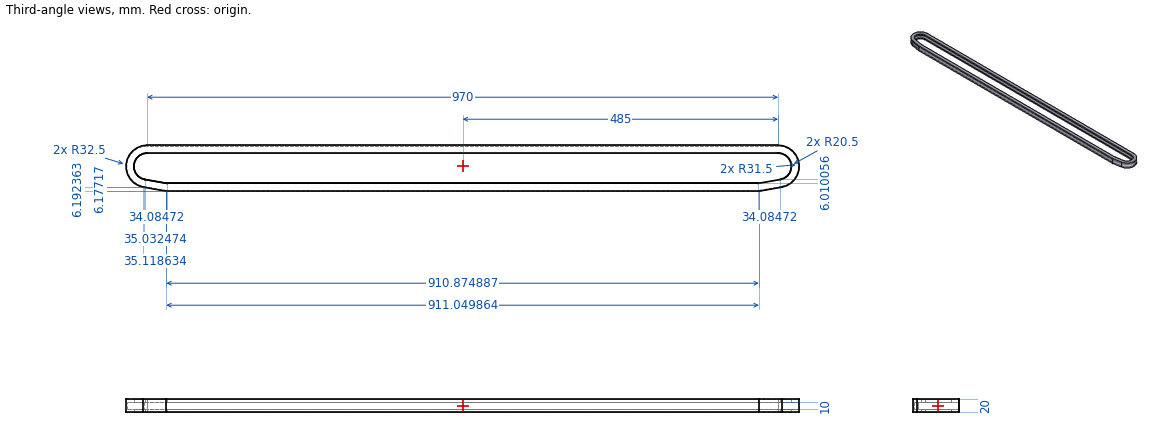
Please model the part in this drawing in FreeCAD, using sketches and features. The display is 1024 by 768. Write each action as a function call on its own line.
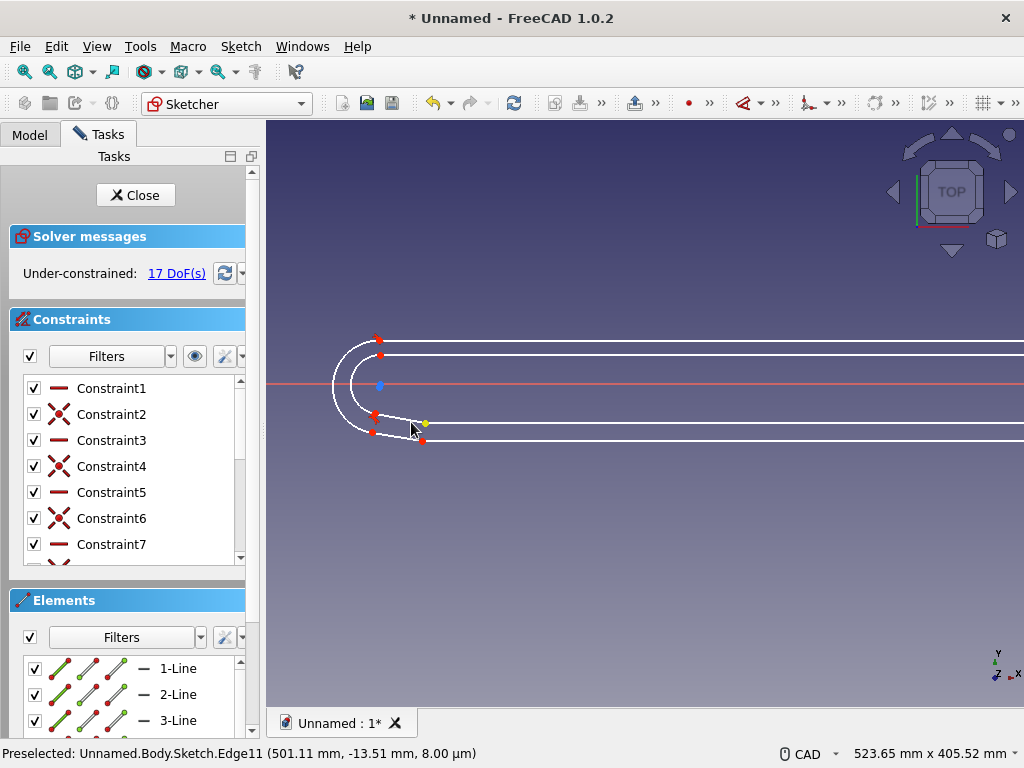
click(410, 420)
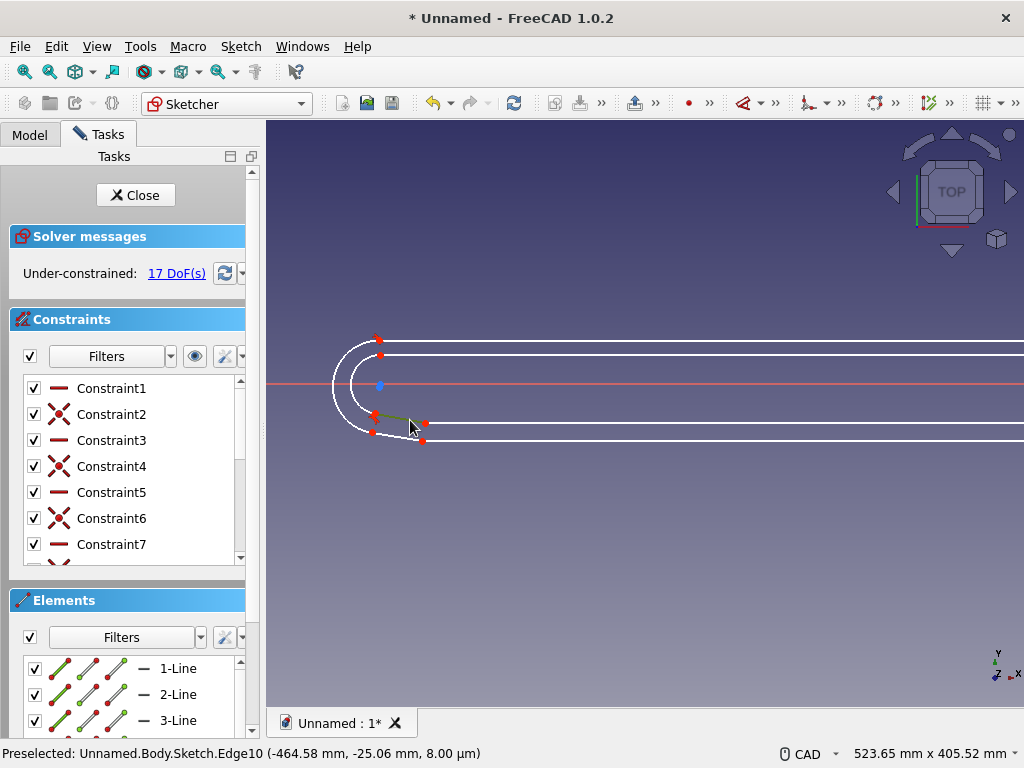
click(358, 366)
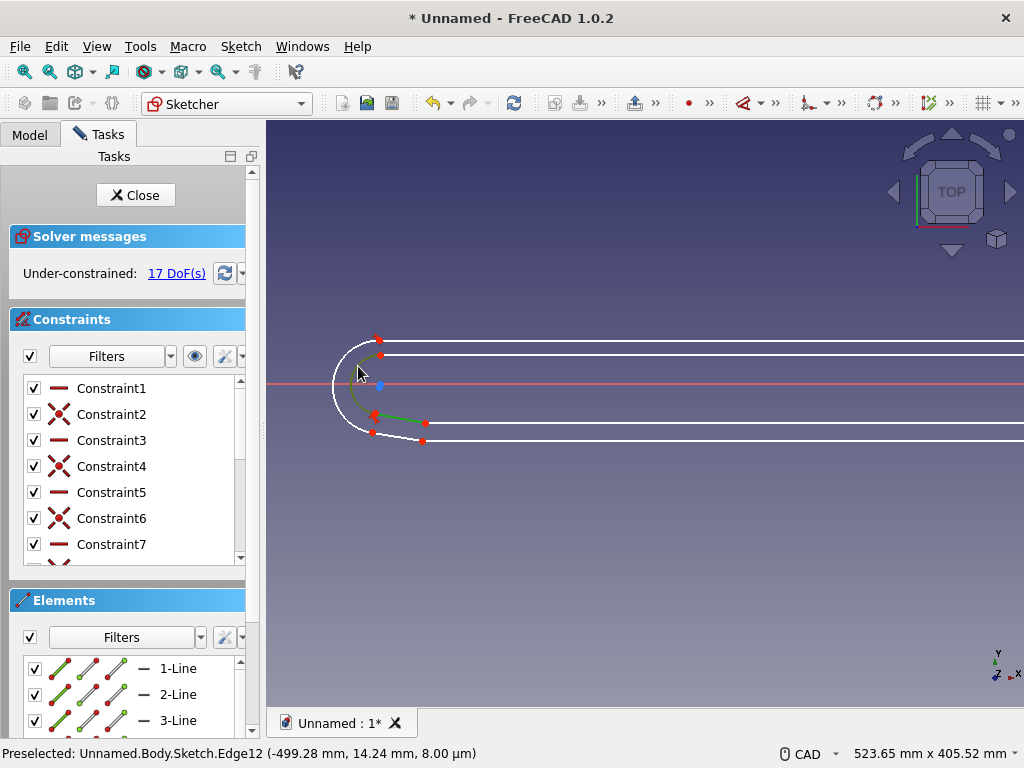
key(t)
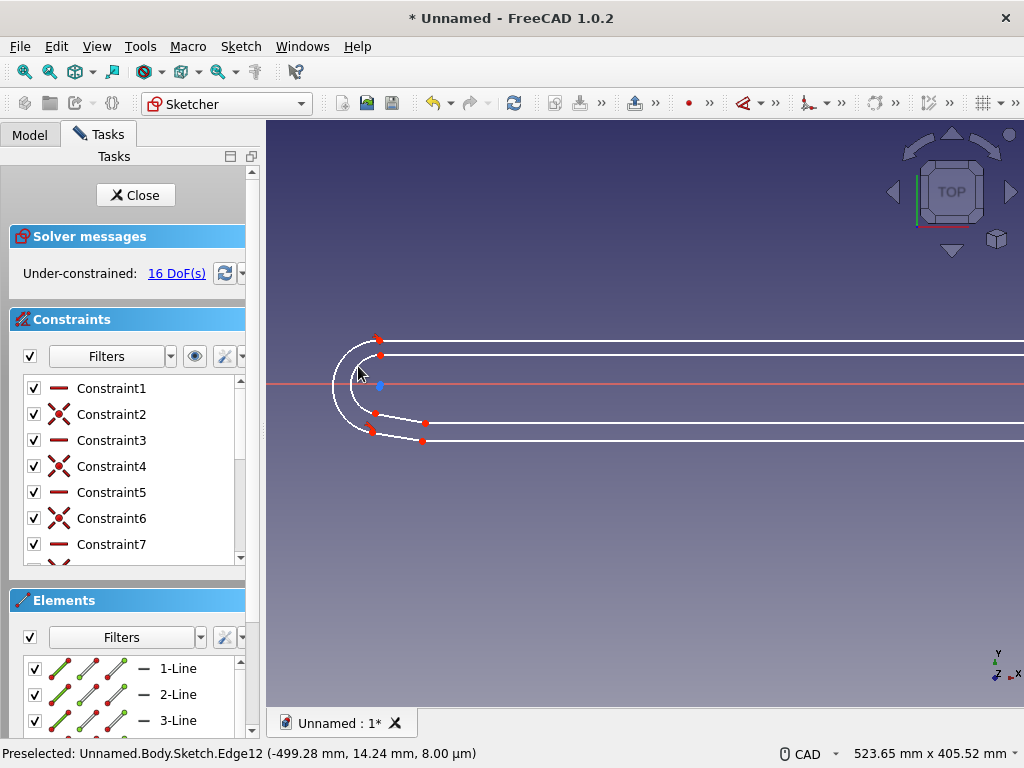
scroll(411, 422, down, 7)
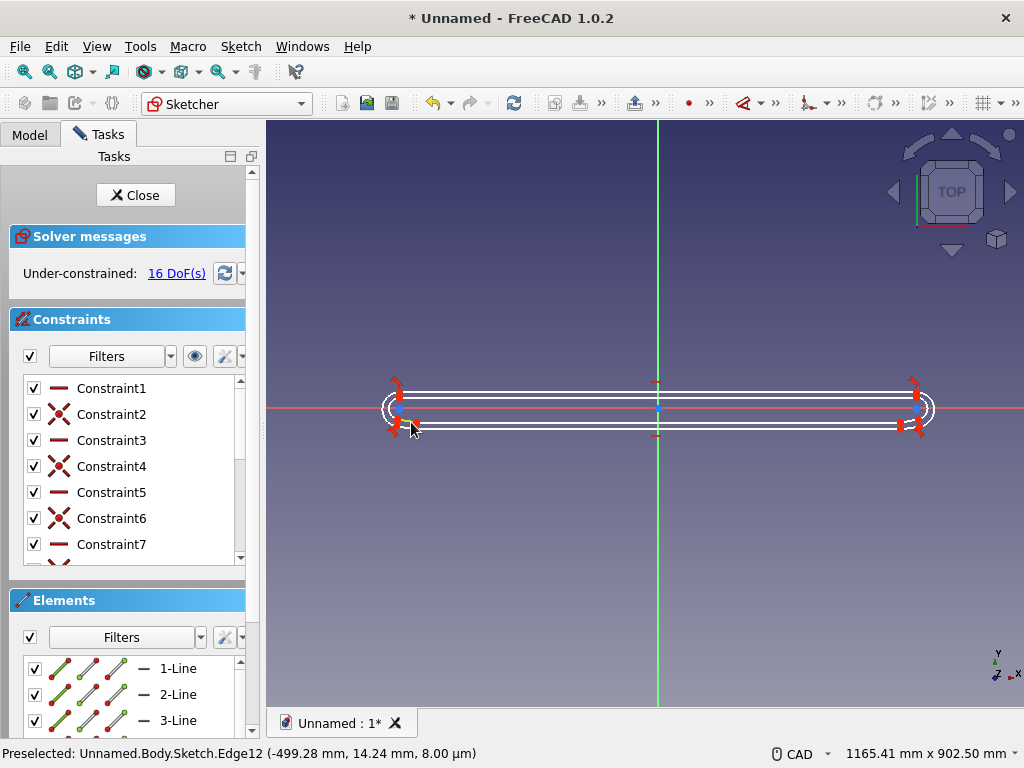
scroll(760, 420, up, 6)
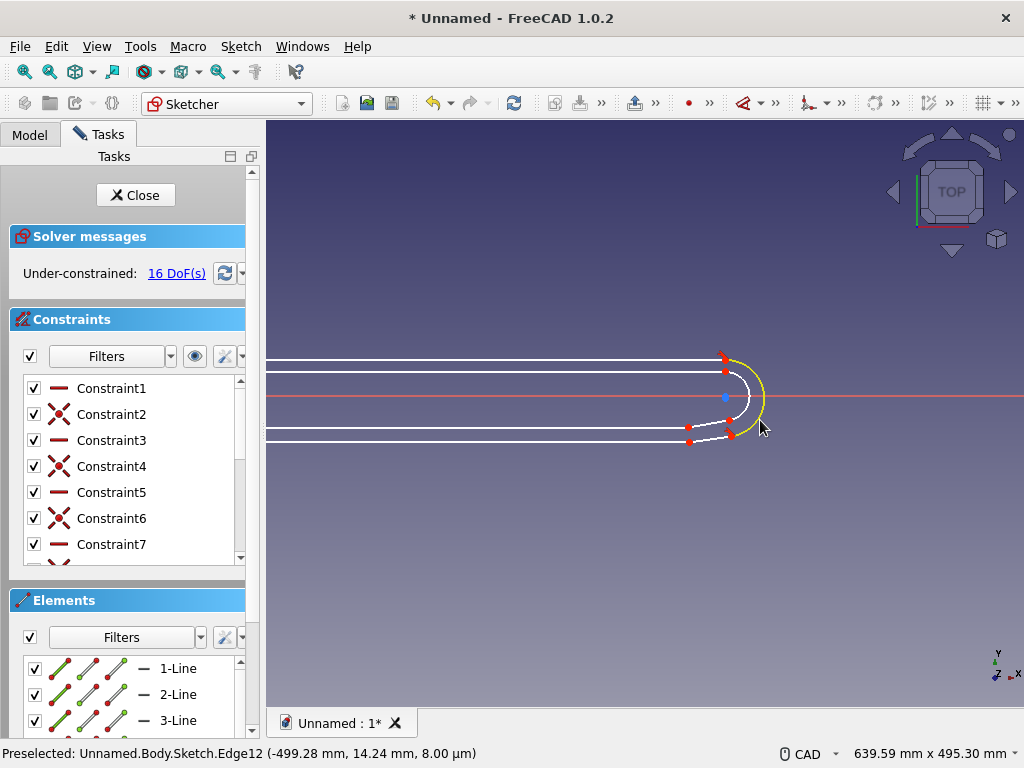
click(759, 418)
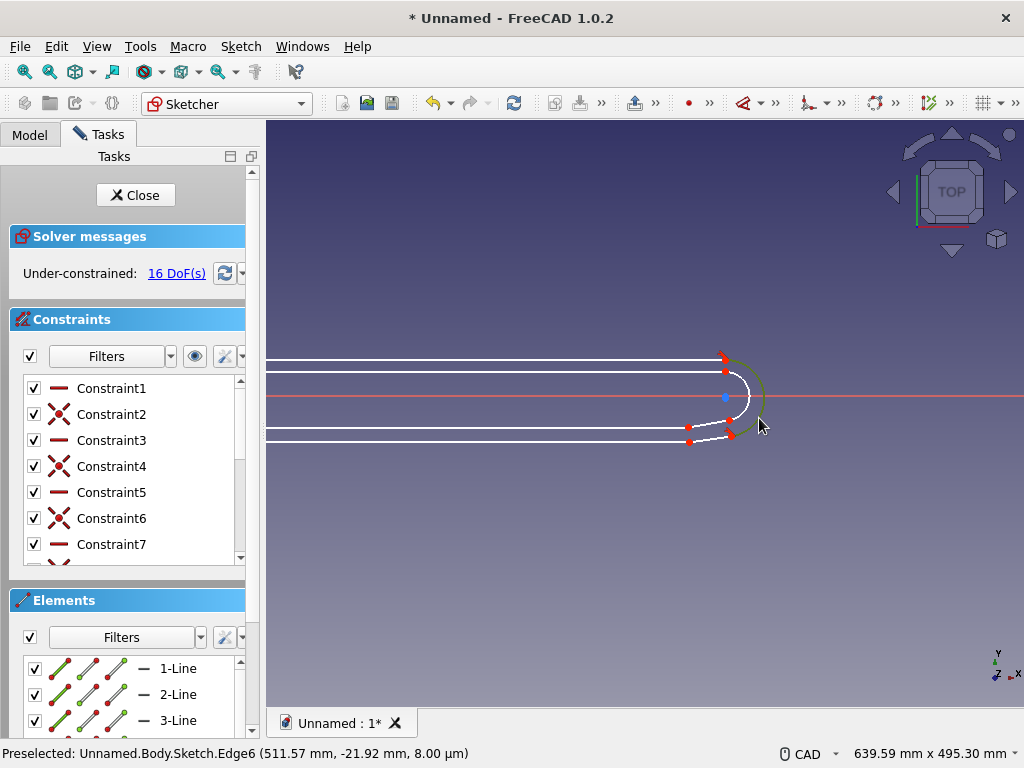
click(746, 408)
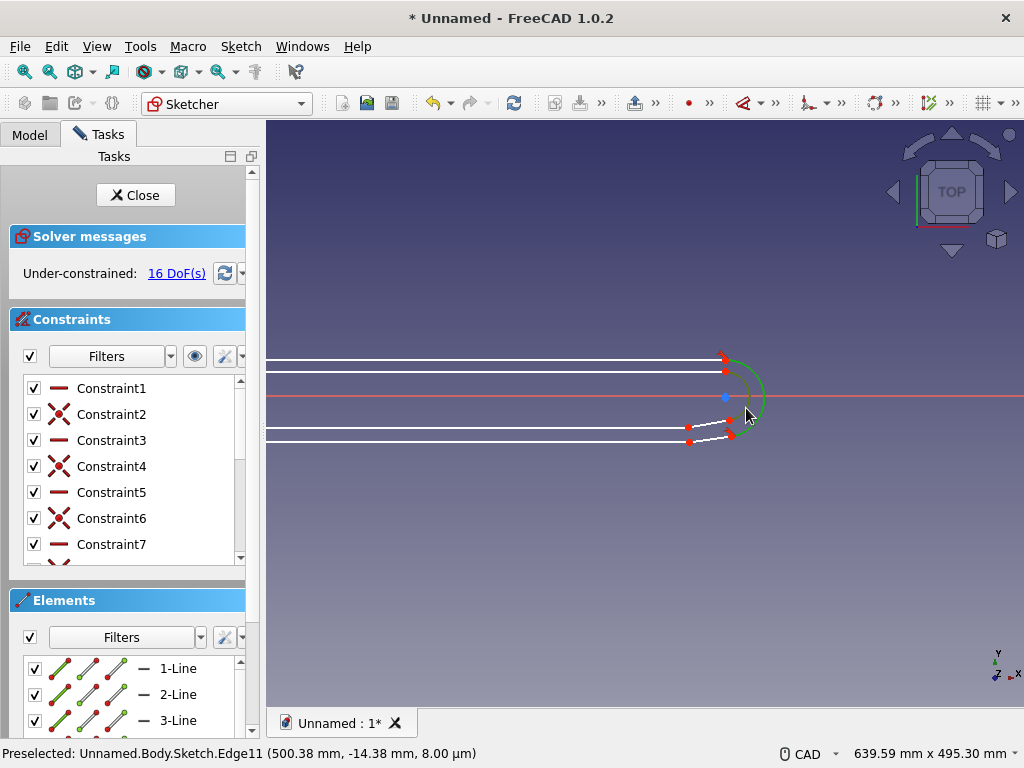
key(c)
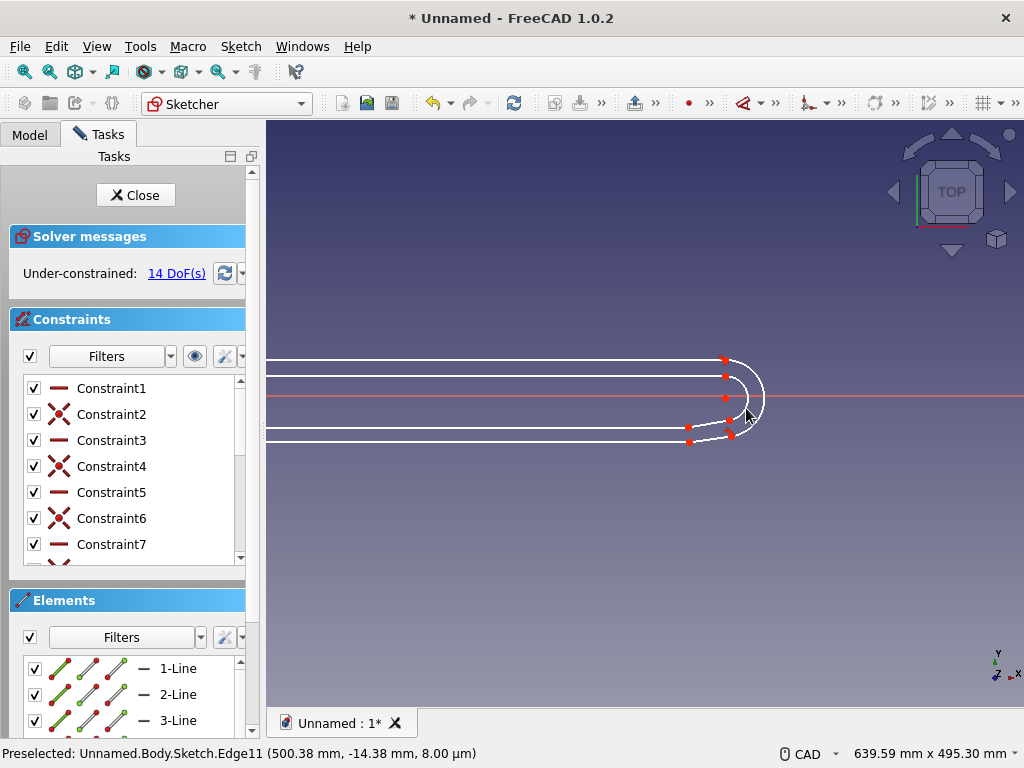
scroll(760, 420, down, 6)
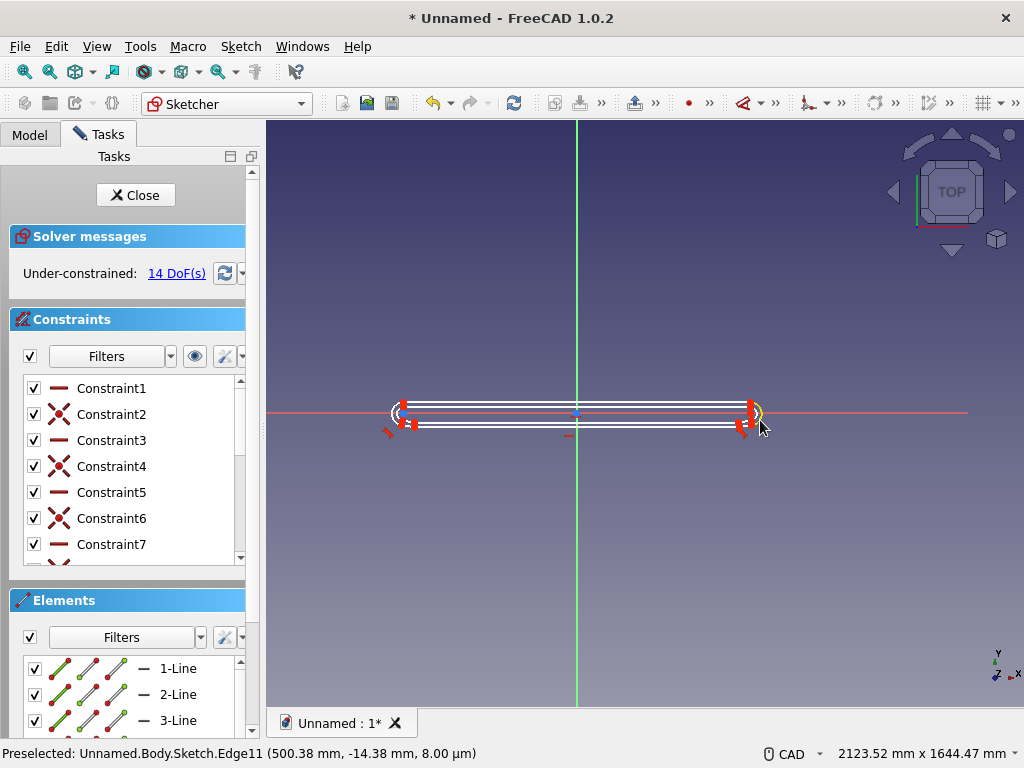
scroll(394, 407, up, 6)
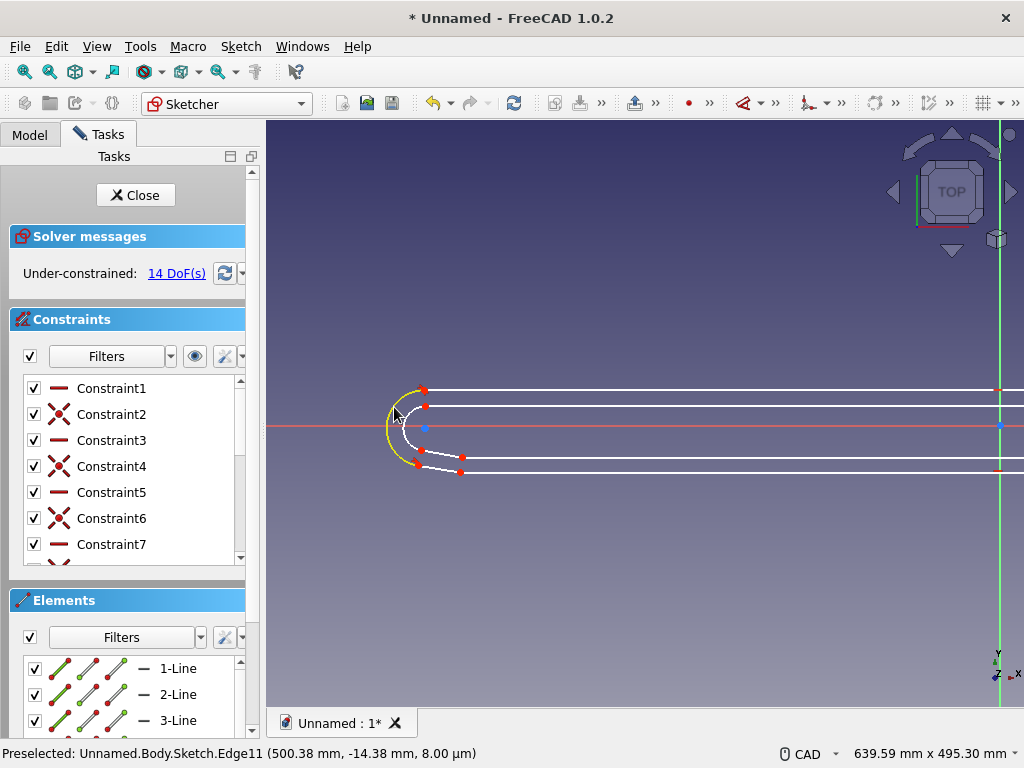
click(395, 404)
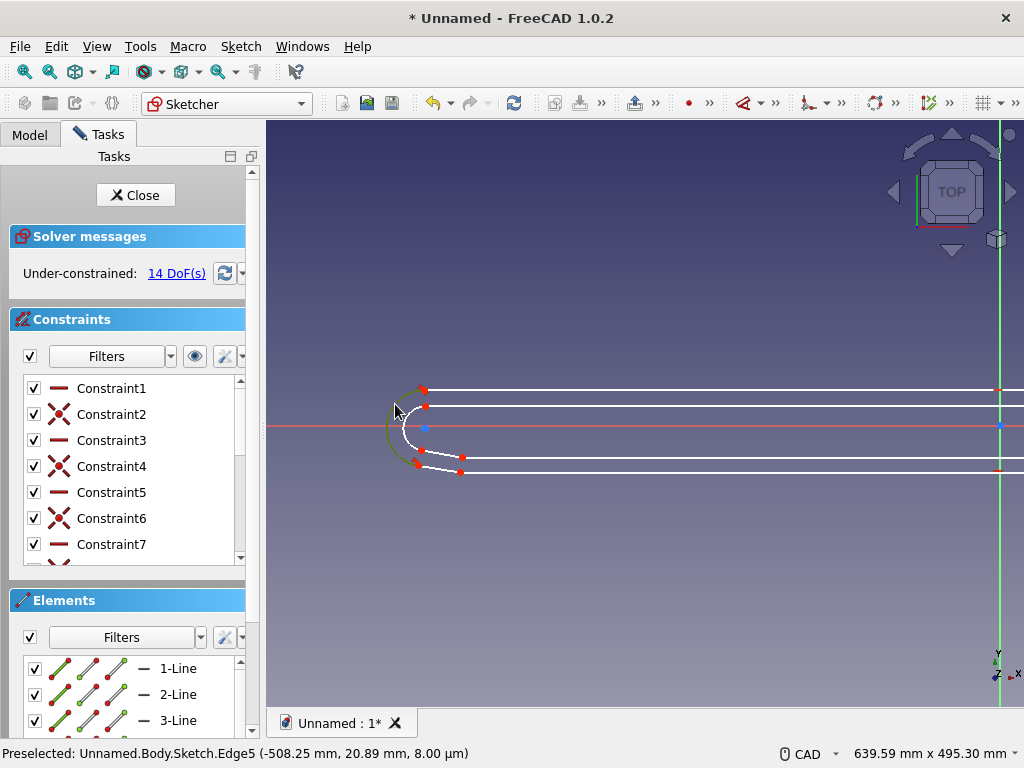
scroll(408, 415, up, 2)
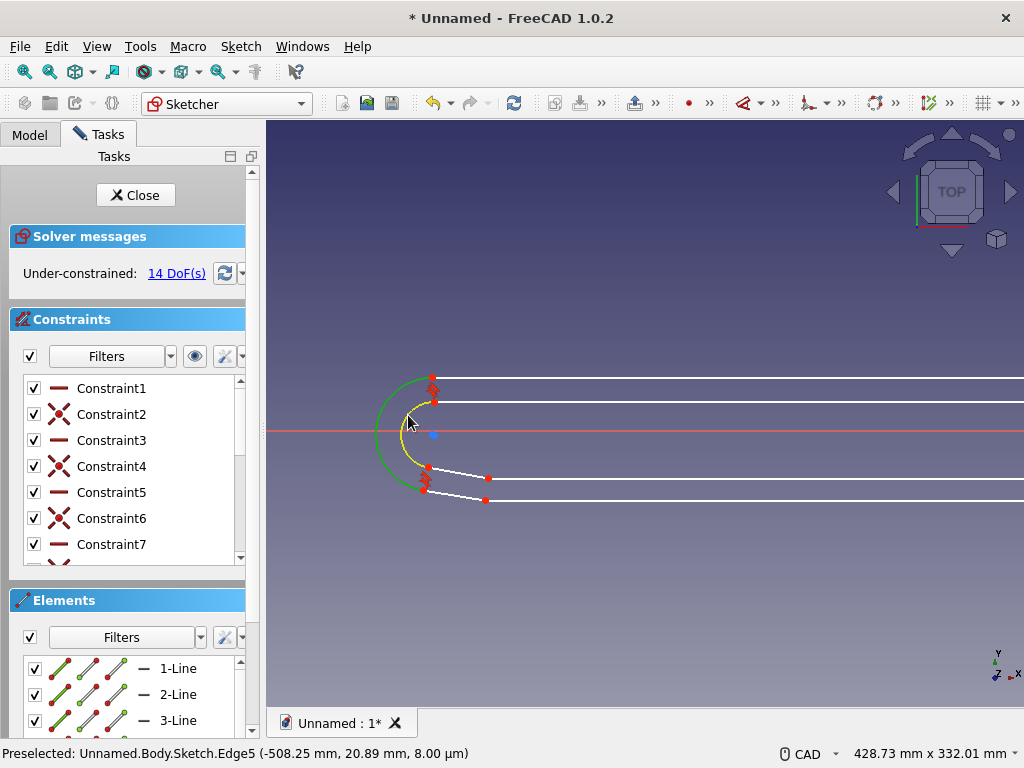
click(409, 414)